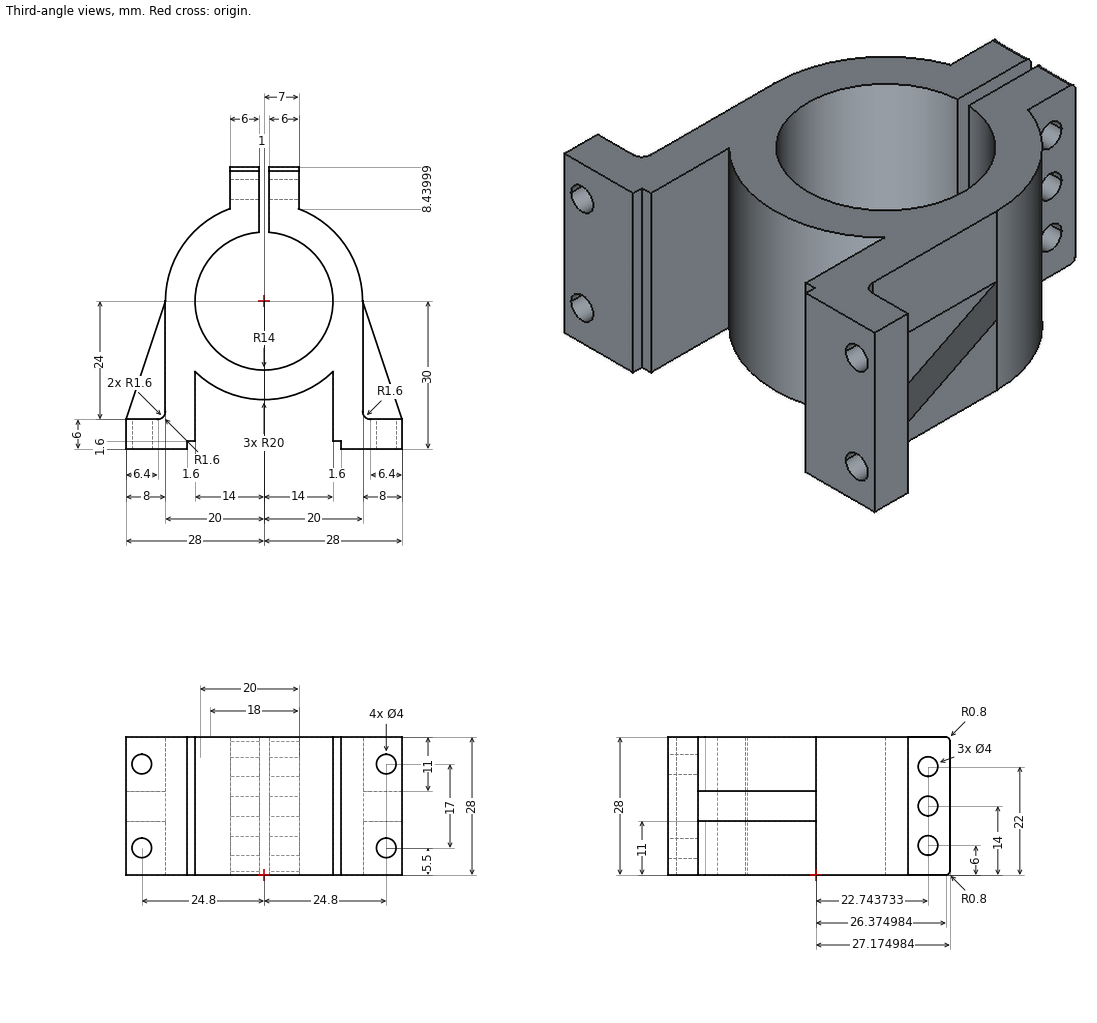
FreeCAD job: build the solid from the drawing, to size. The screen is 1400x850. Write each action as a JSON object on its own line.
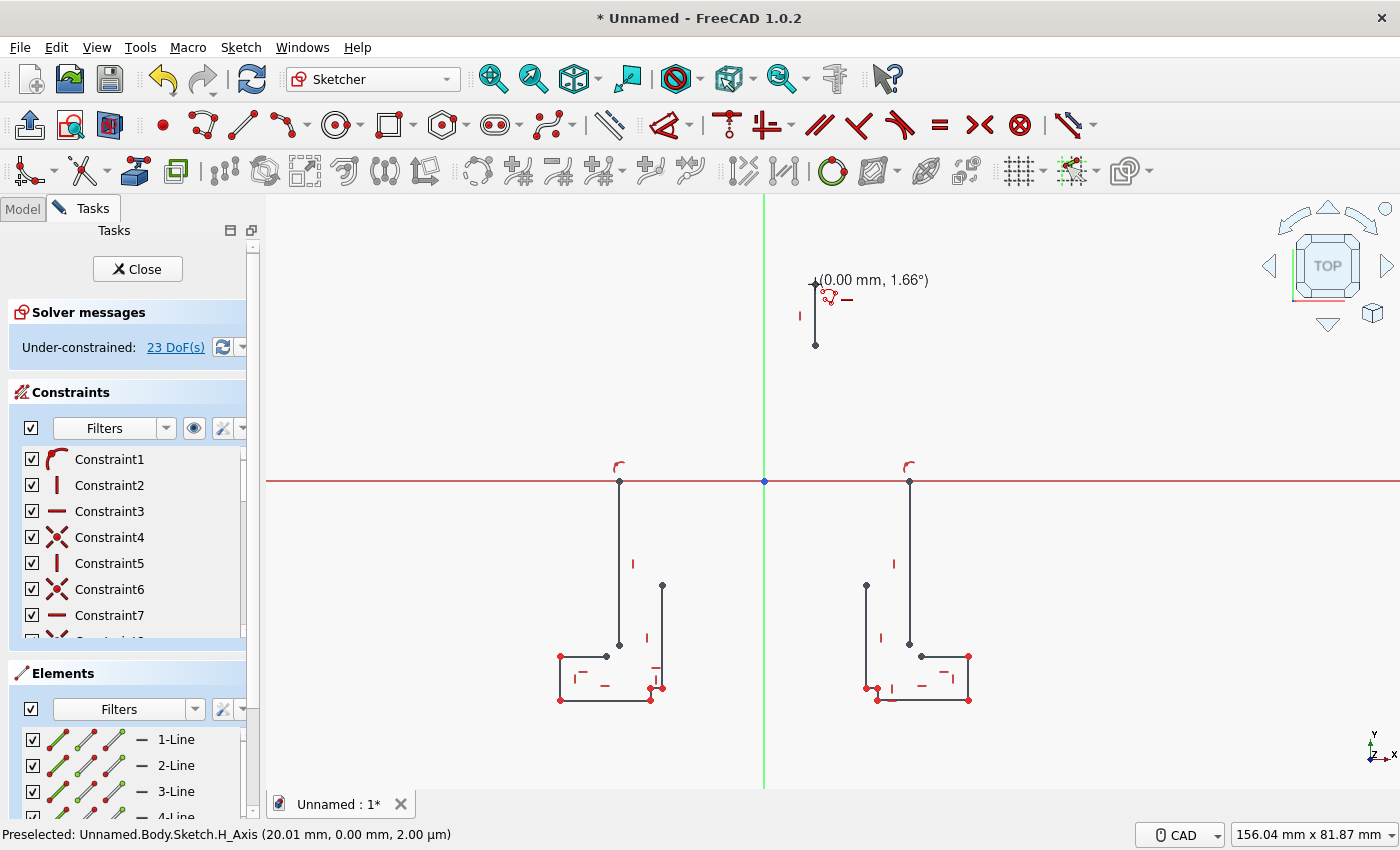
{"action": "scroll", "coordinate": [772, 284], "scroll_direction": "up", "scroll_amount": 4}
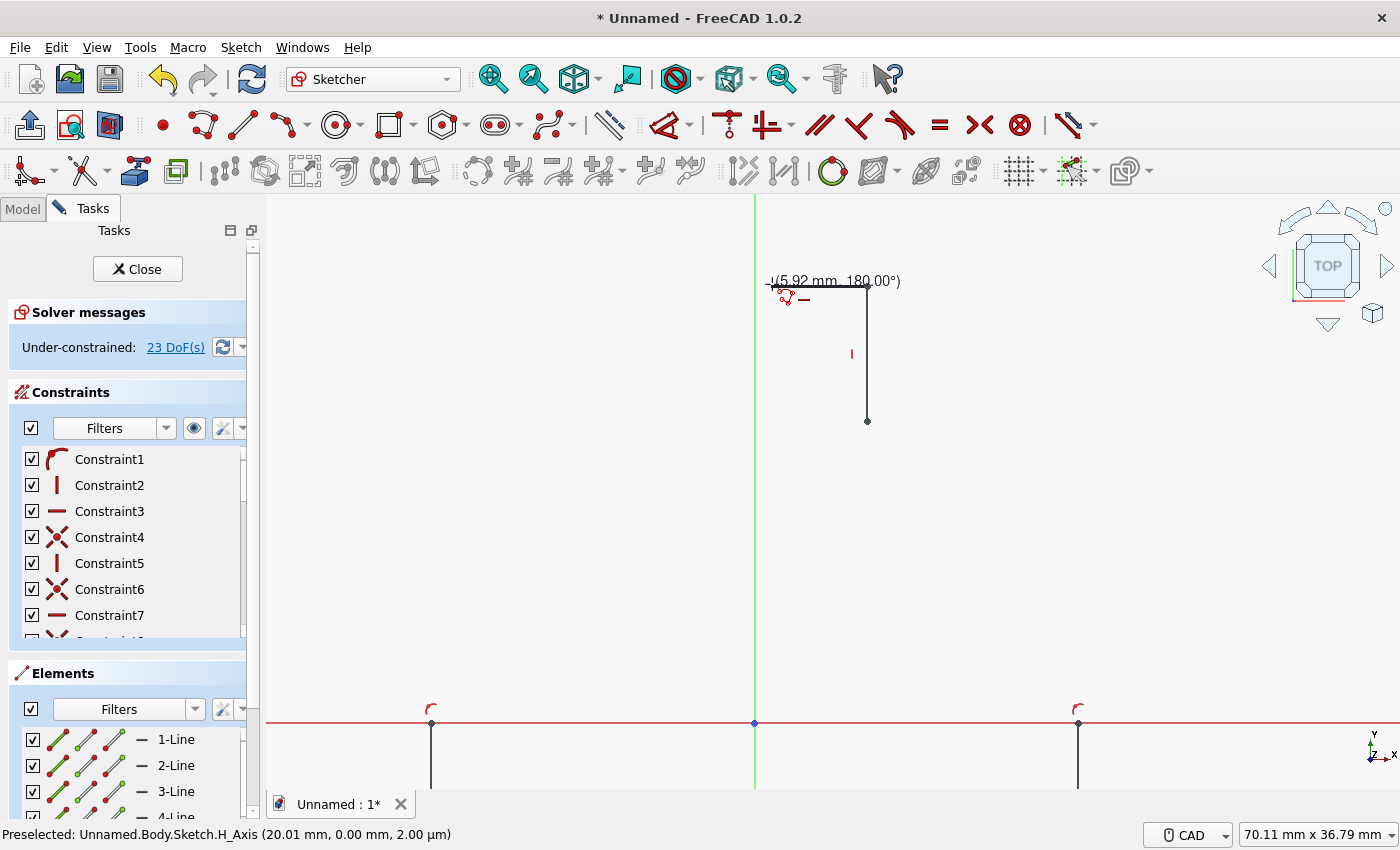
{"action": "left_click", "coordinate": [771, 284]}
{"action": "left_click", "coordinate": [771, 497]}
{"action": "right_click", "coordinate": [771, 497]}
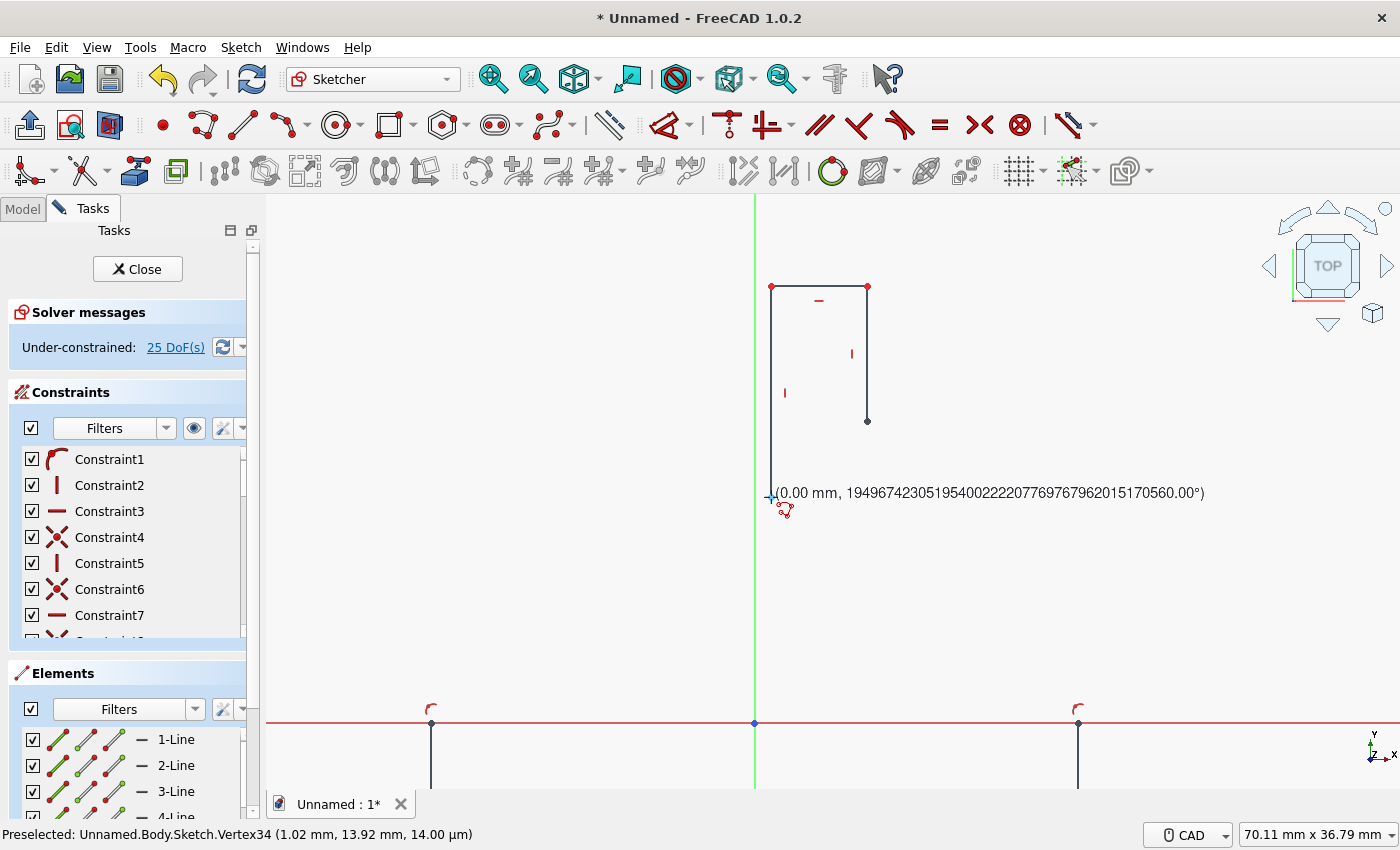
{"action": "left_click", "coordinate": [738, 497]}
{"action": "left_click", "coordinate": [738, 284]}
{"action": "left_click", "coordinate": [641, 284]}
{"action": "left_click", "coordinate": [641, 420]}
{"action": "right_click", "coordinate": [641, 420]}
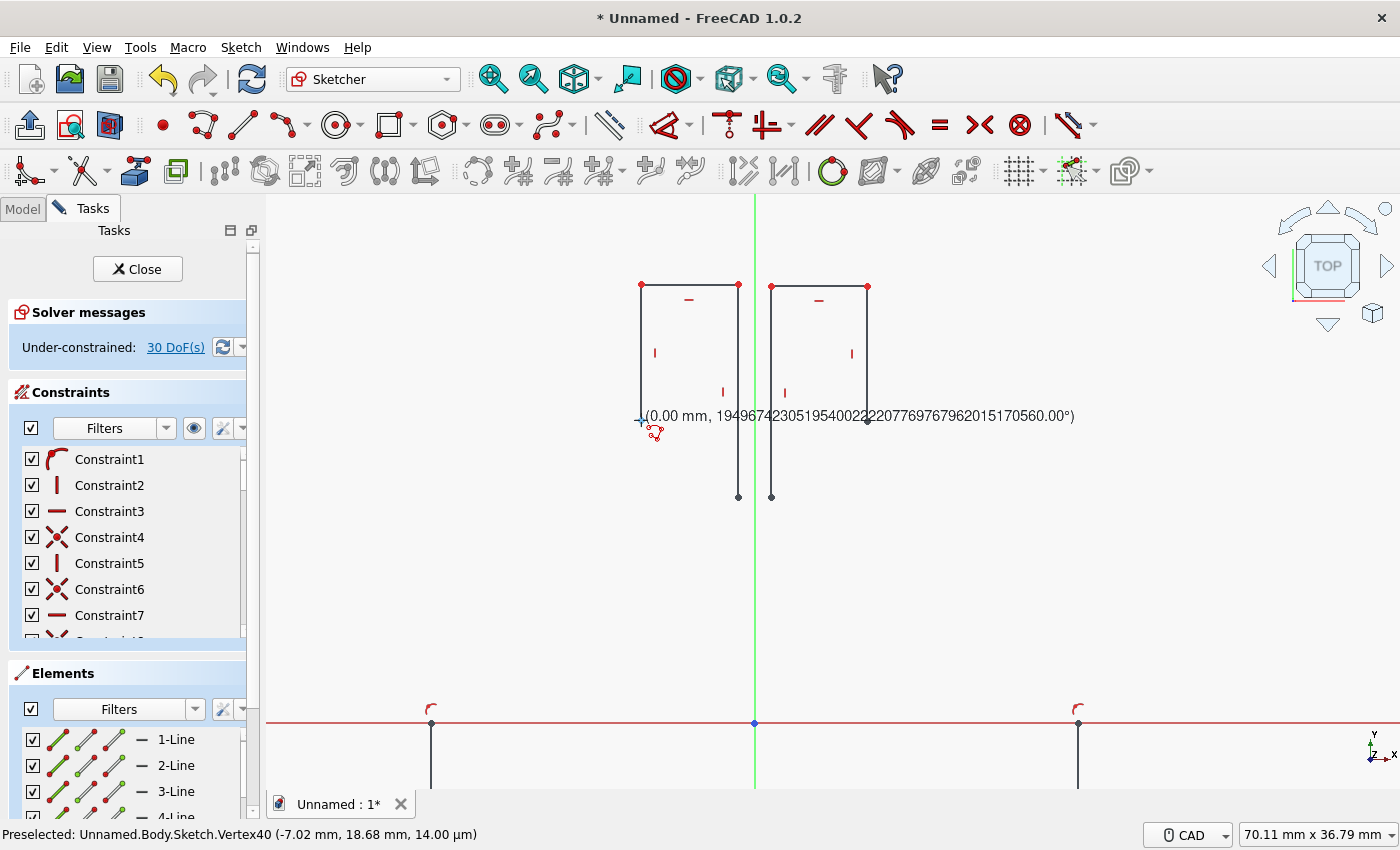
{"action": "left_click", "coordinate": [284, 126]}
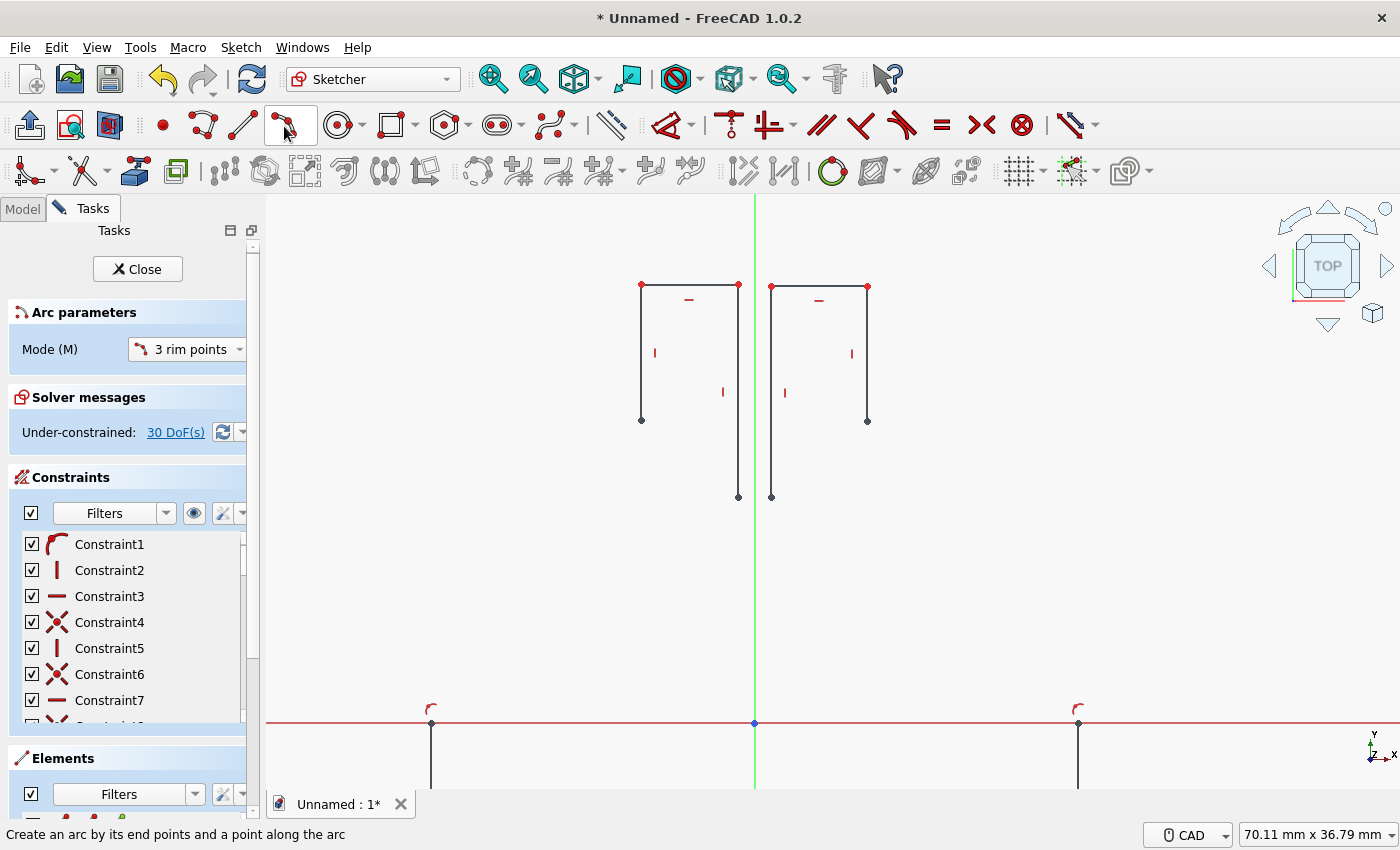
{"action": "scroll", "coordinate": [773, 284], "scroll_direction": "down", "scroll_amount": 4}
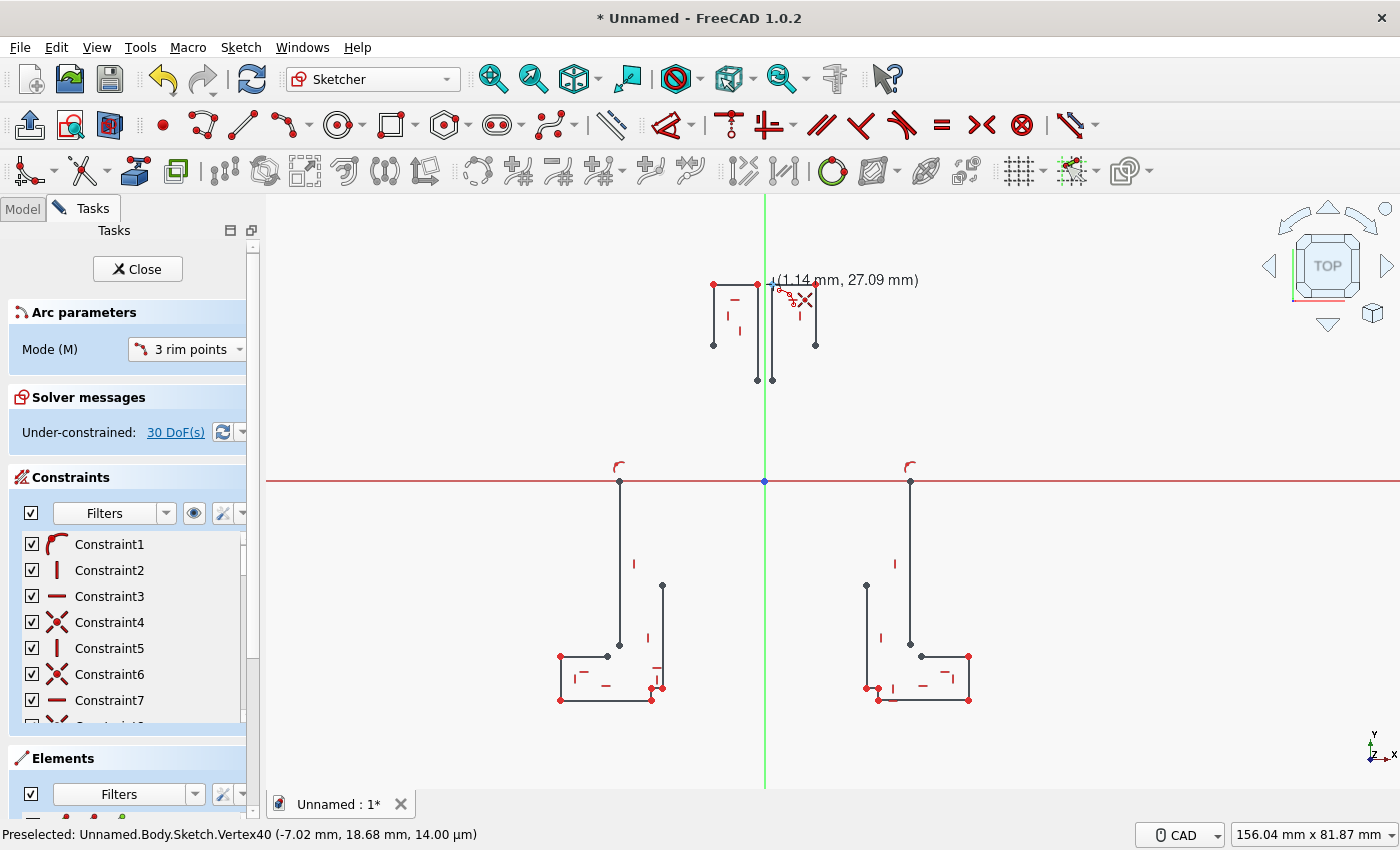
{"action": "left_click", "coordinate": [620, 646]}
{"action": "left_click", "coordinate": [607, 657]}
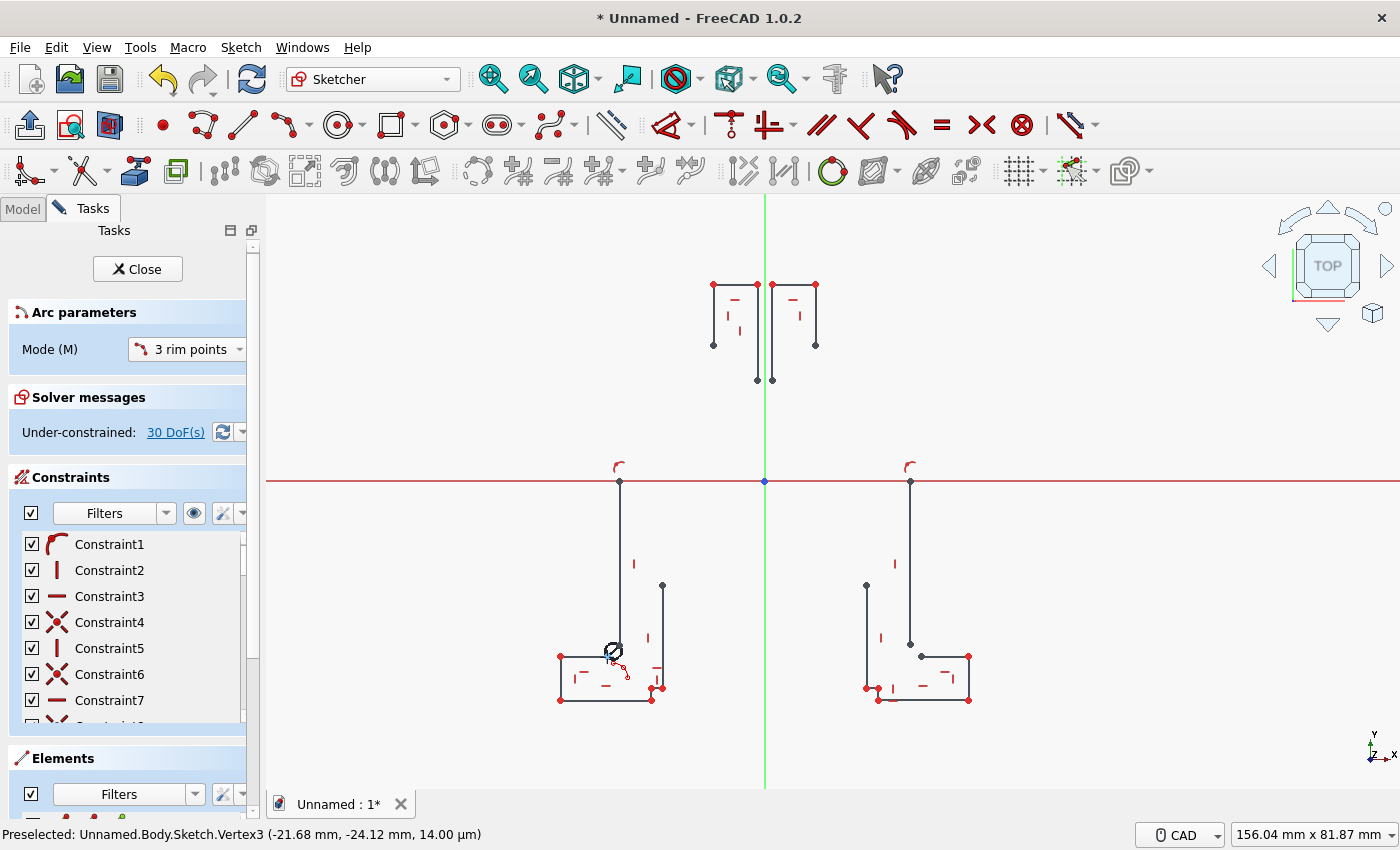
{"action": "scroll", "coordinate": [616, 652], "scroll_direction": "up", "scroll_amount": 8}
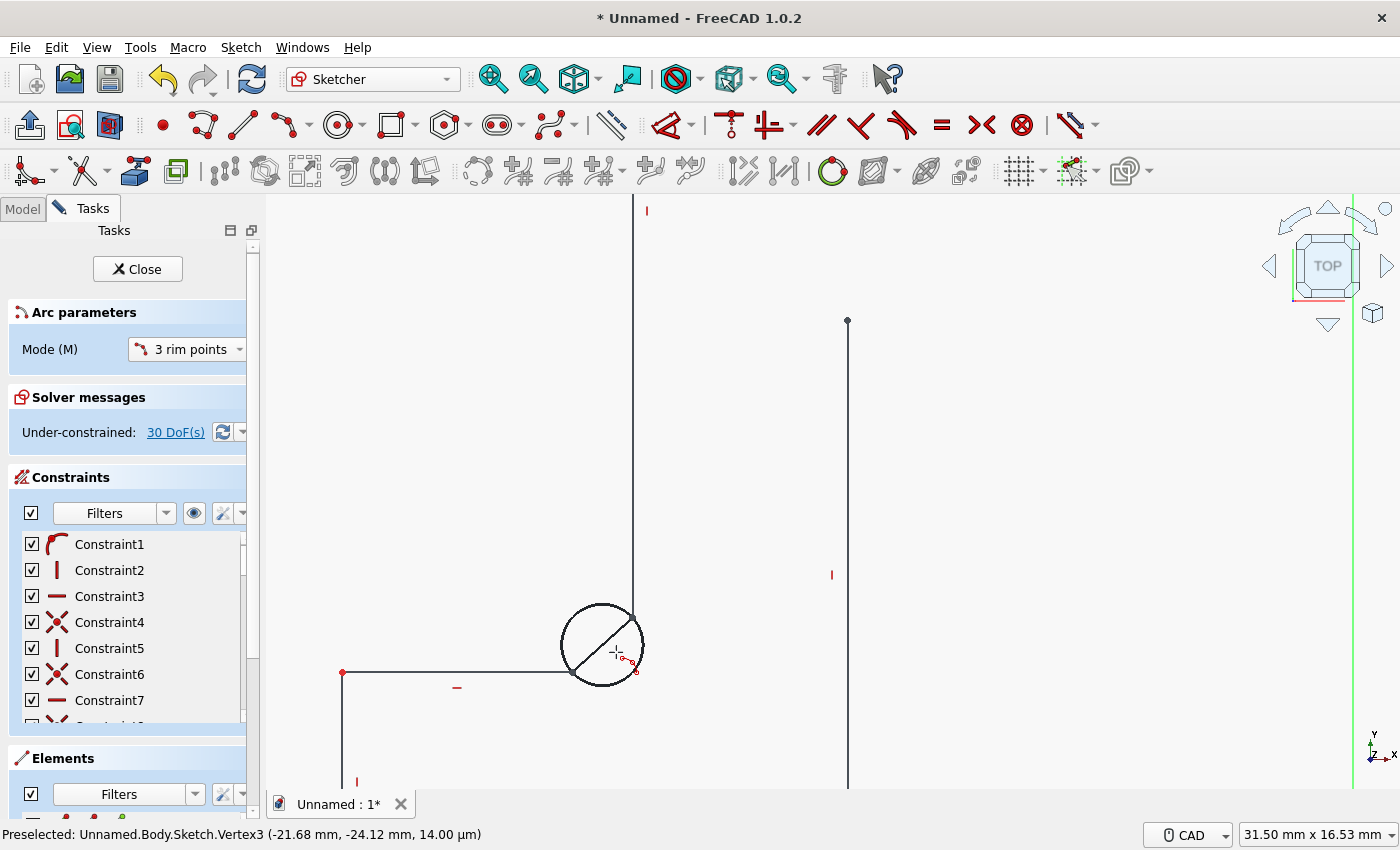
{"action": "left_click", "coordinate": [616, 651]}